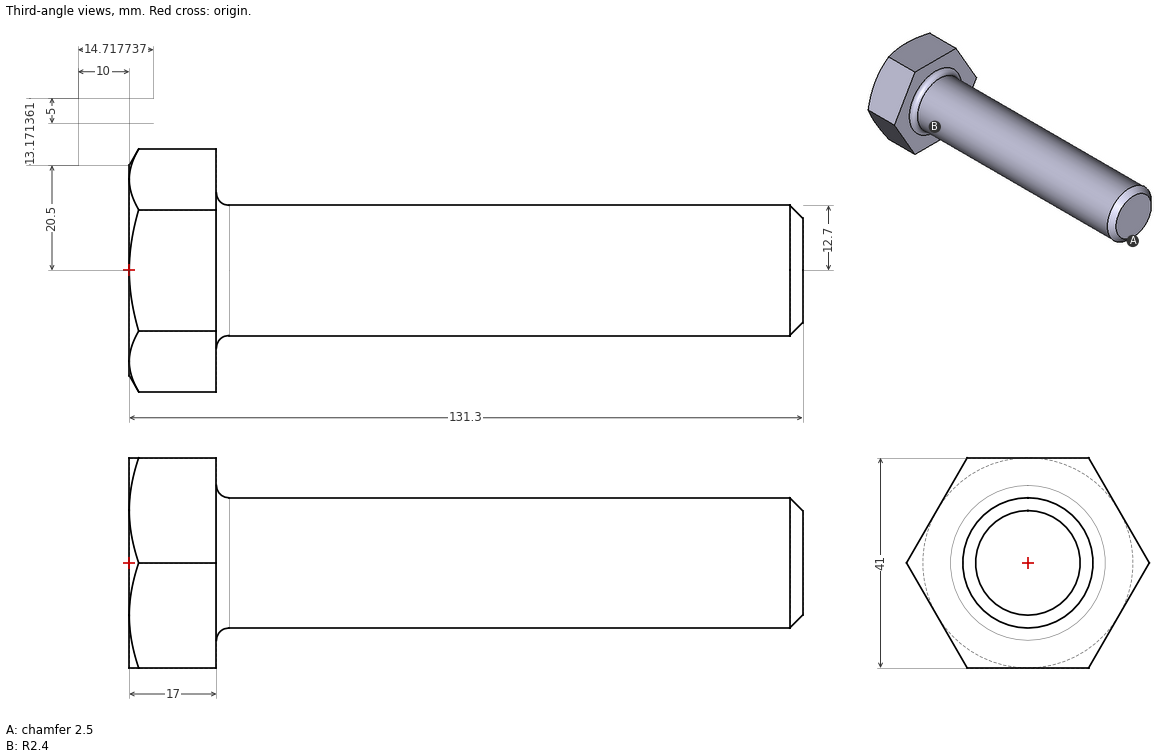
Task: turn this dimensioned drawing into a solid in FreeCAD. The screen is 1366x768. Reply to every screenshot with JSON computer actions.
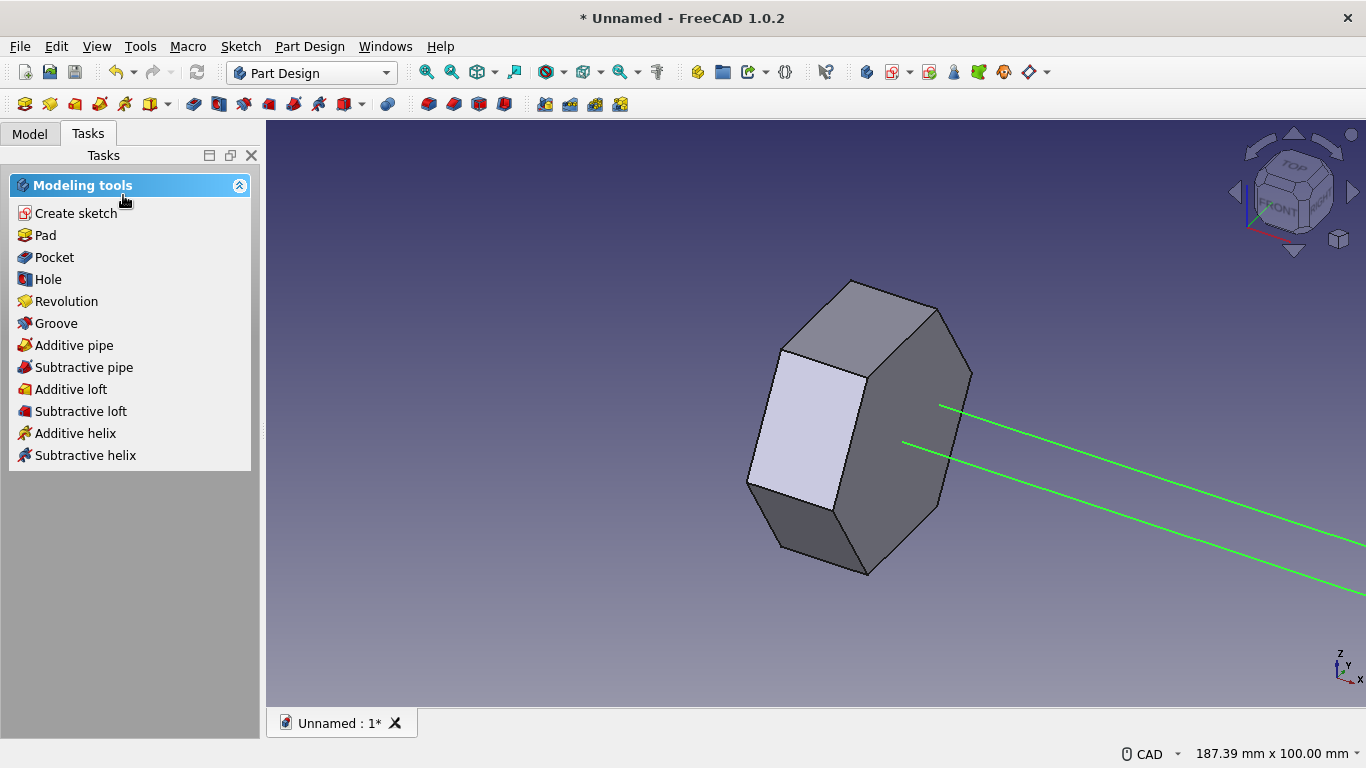
{"action": "left_click", "coordinate": [50, 104]}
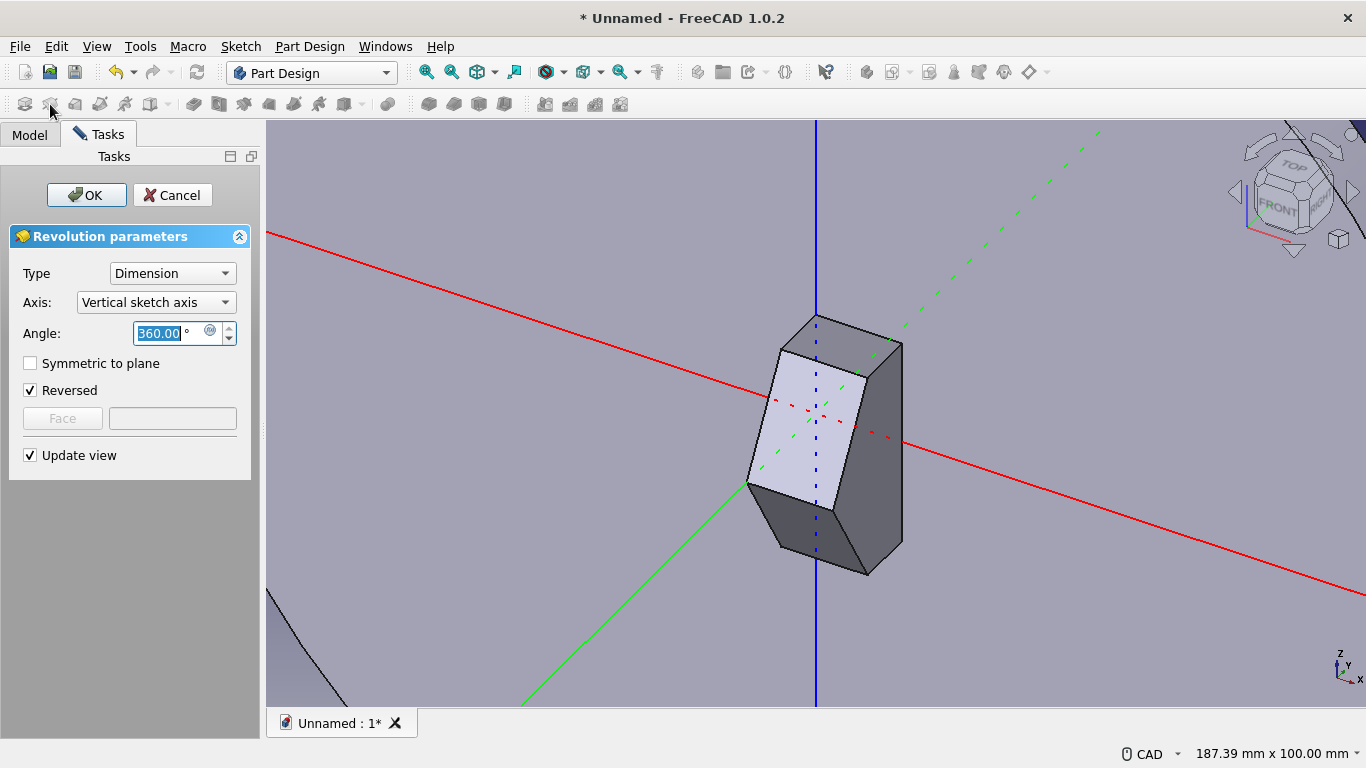
{"action": "left_click", "coordinate": [157, 302]}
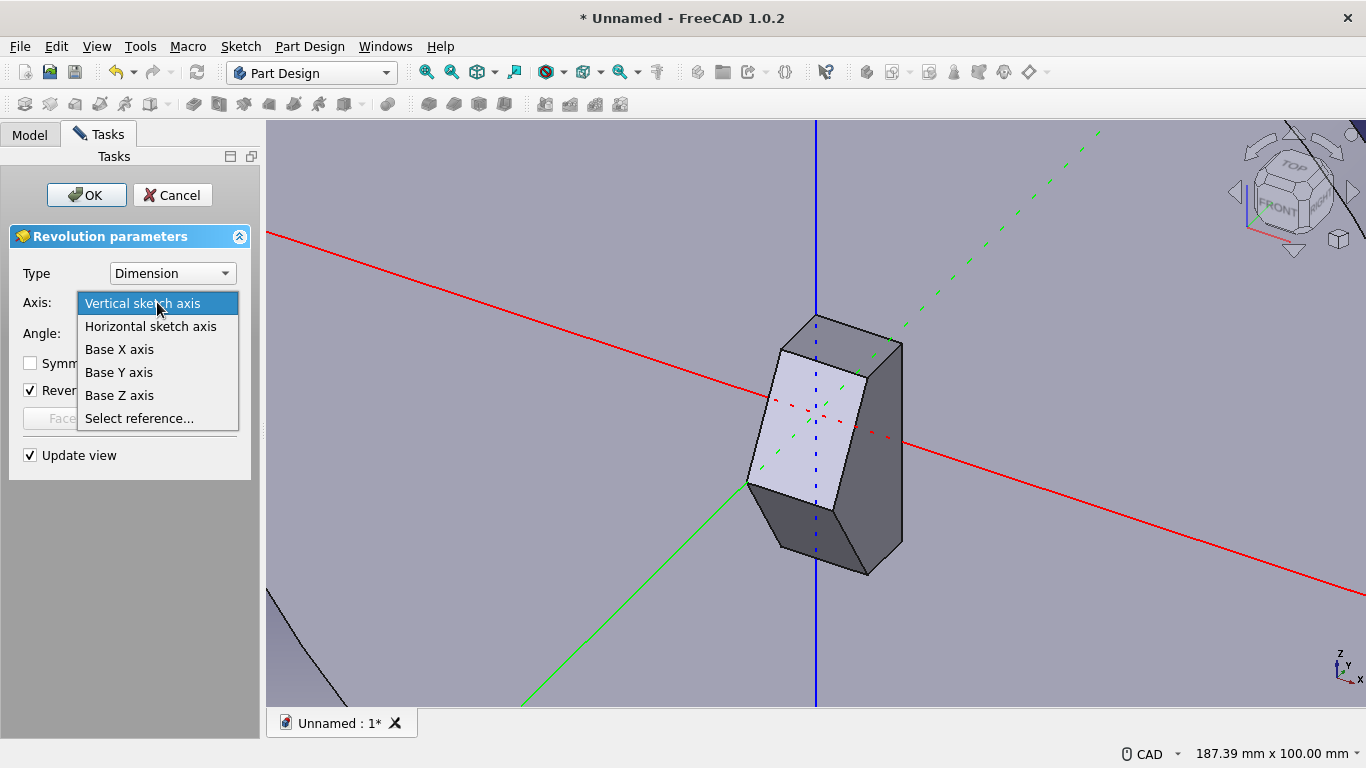
{"action": "left_click", "coordinate": [156, 326]}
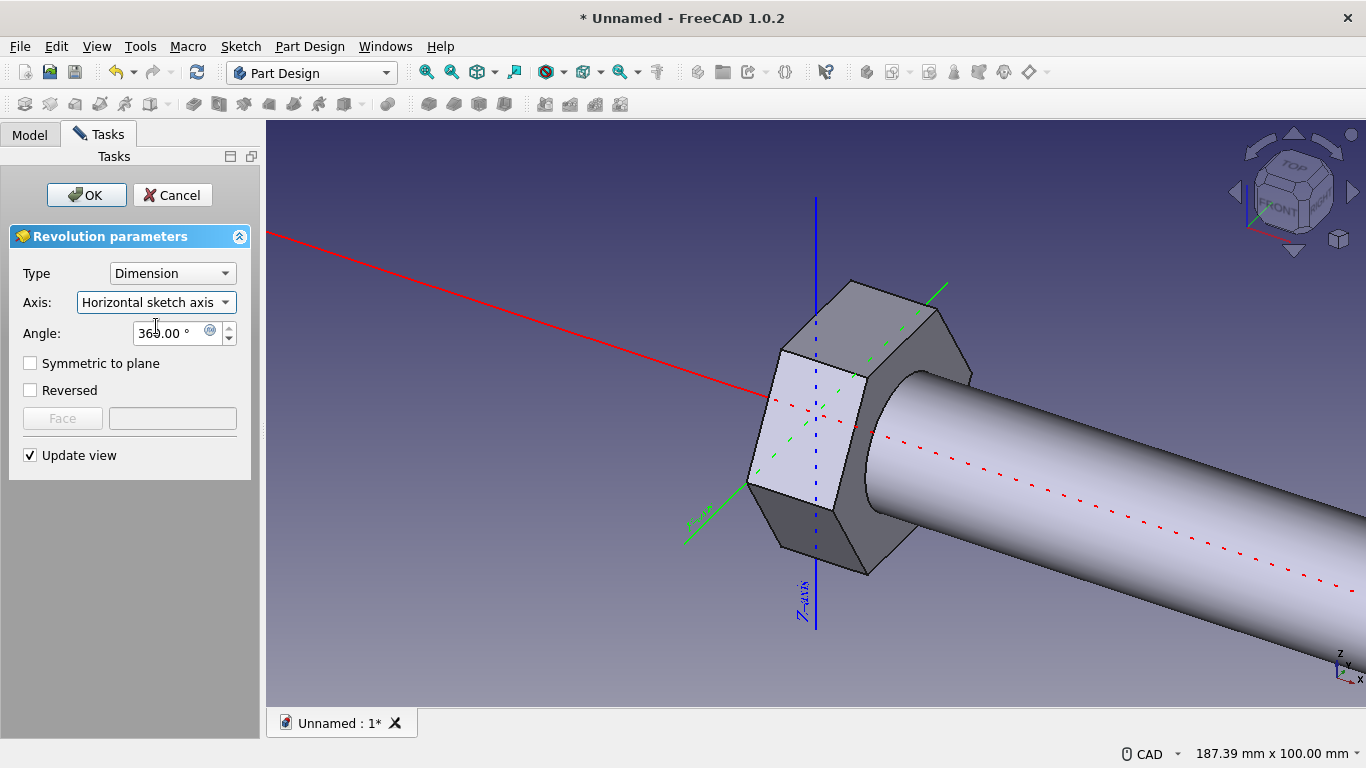
{"action": "left_click", "coordinate": [87, 195]}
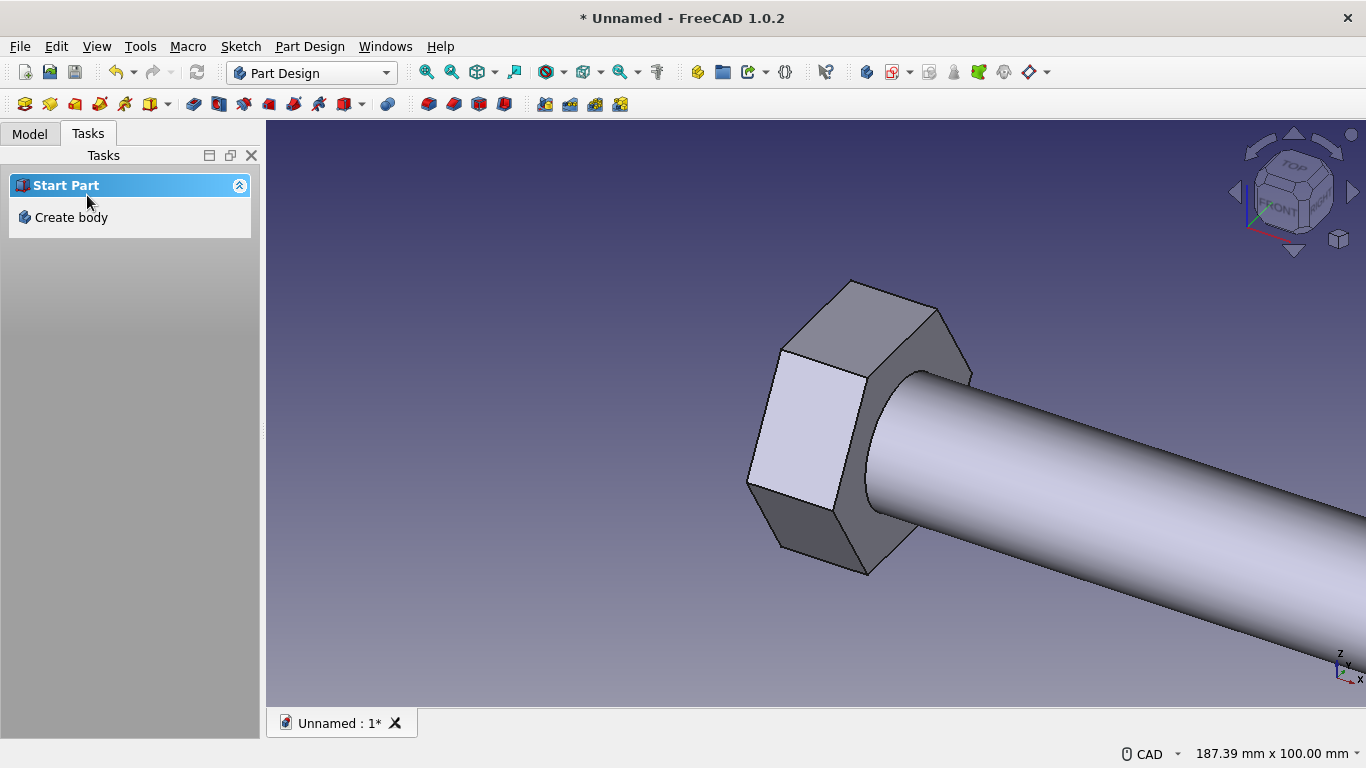
{"action": "key", "text": "v f"}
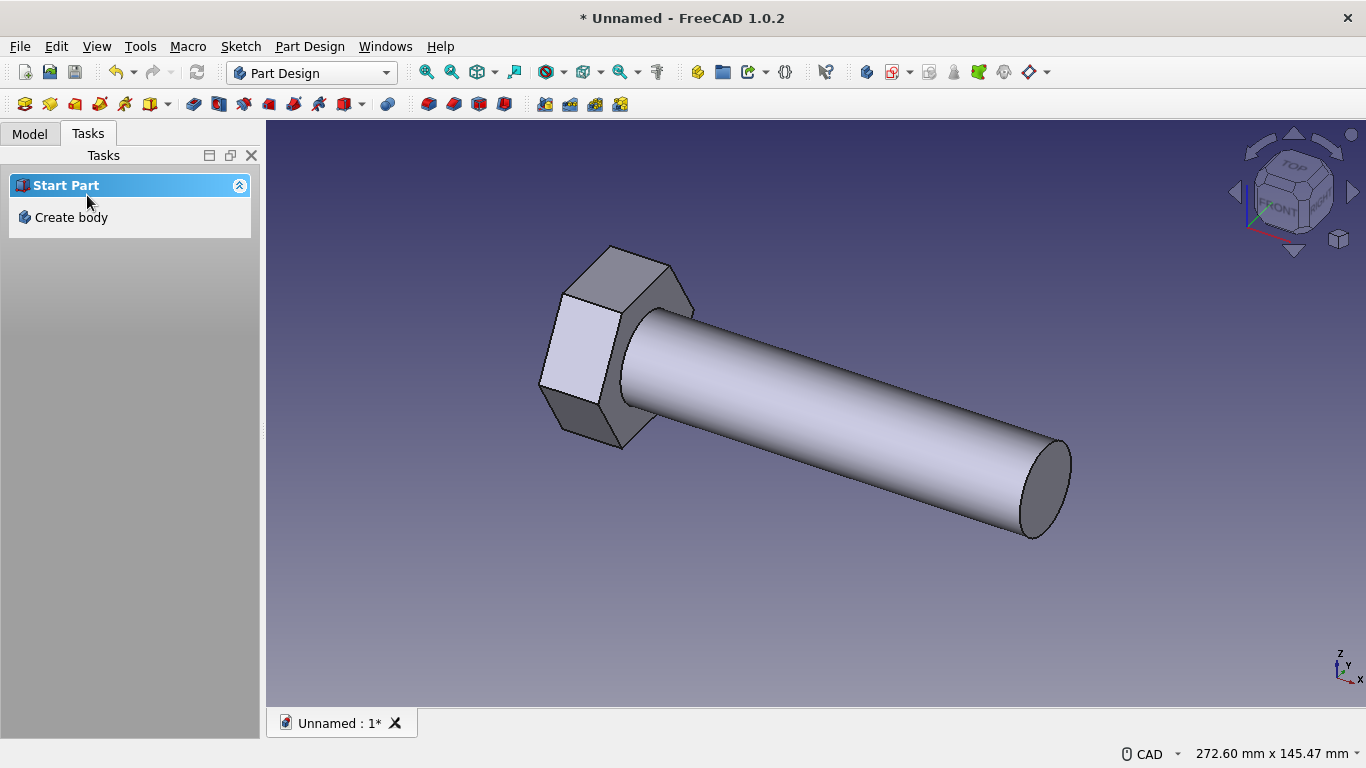
{"action": "left_click", "coordinate": [892, 72]}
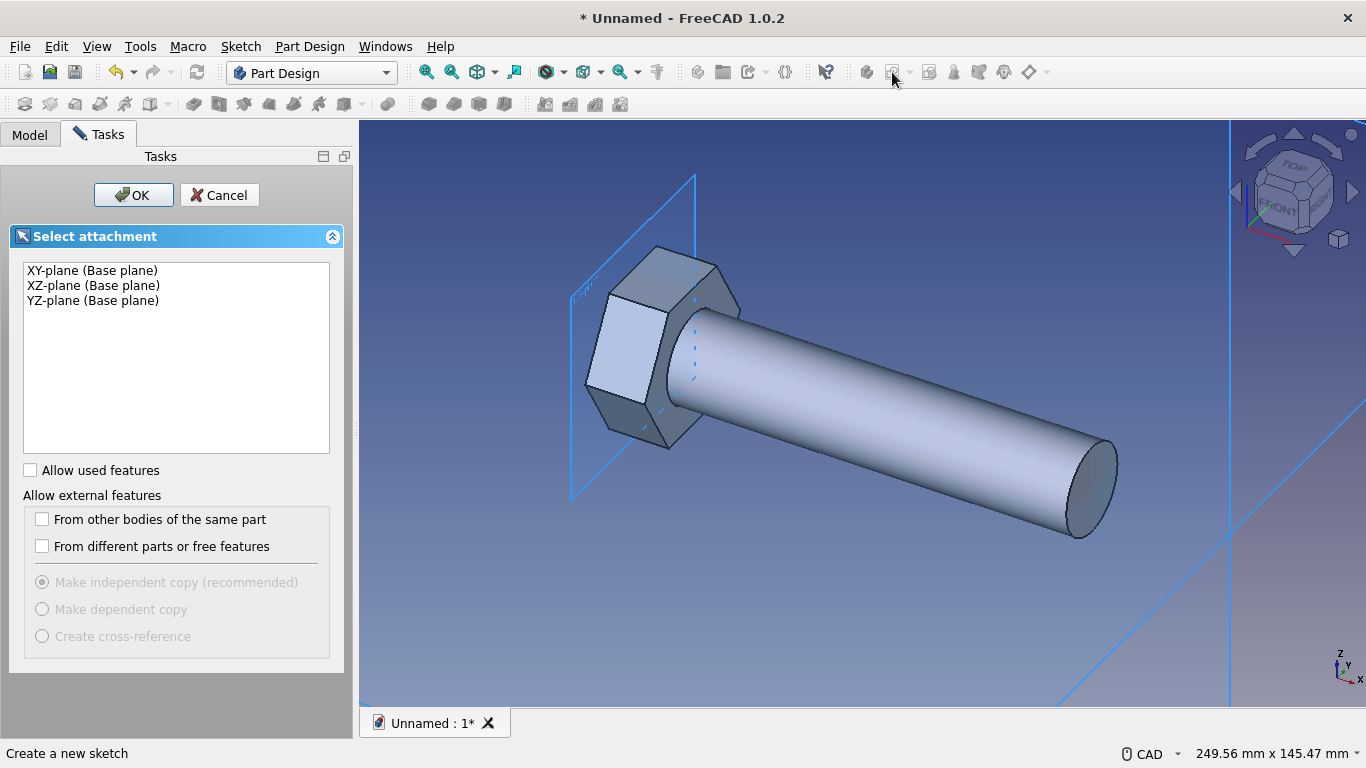
{"action": "left_click", "coordinate": [84, 270]}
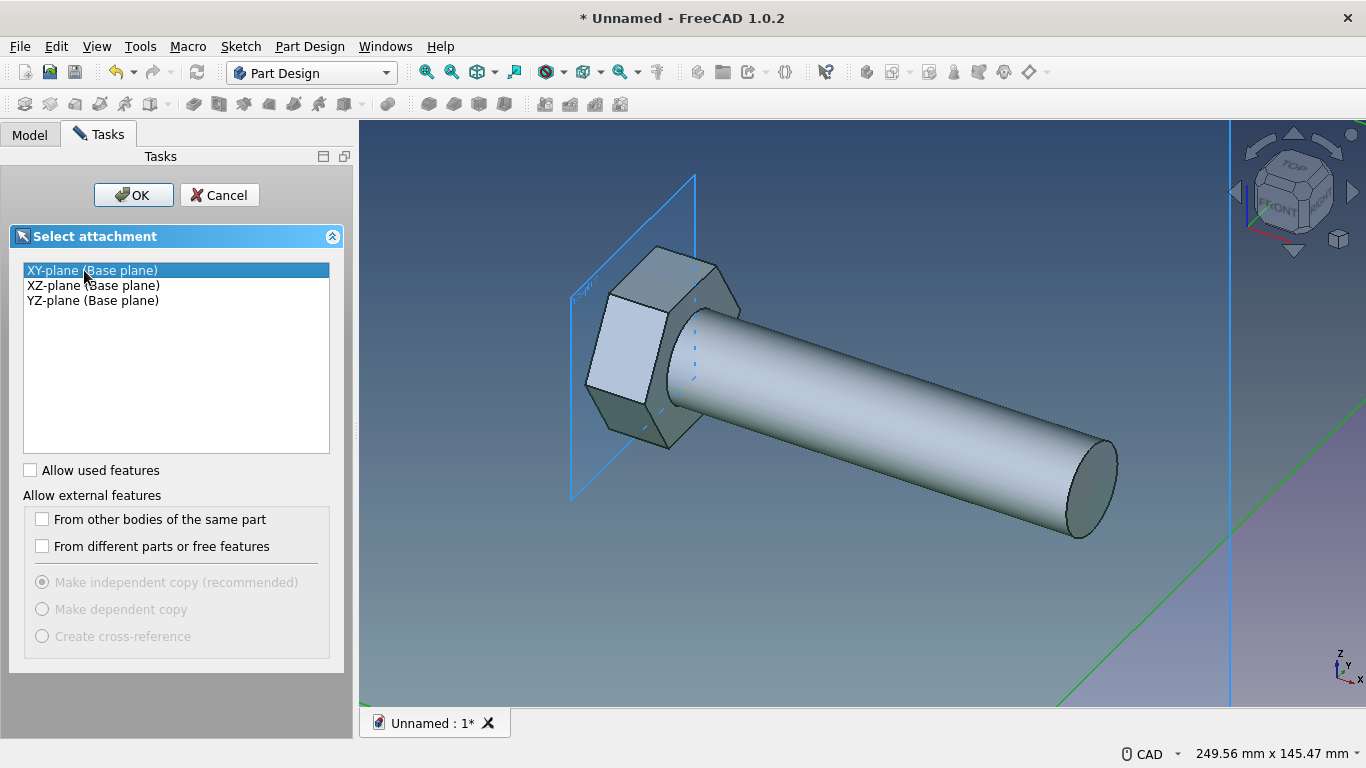
{"action": "left_click", "coordinate": [134, 195]}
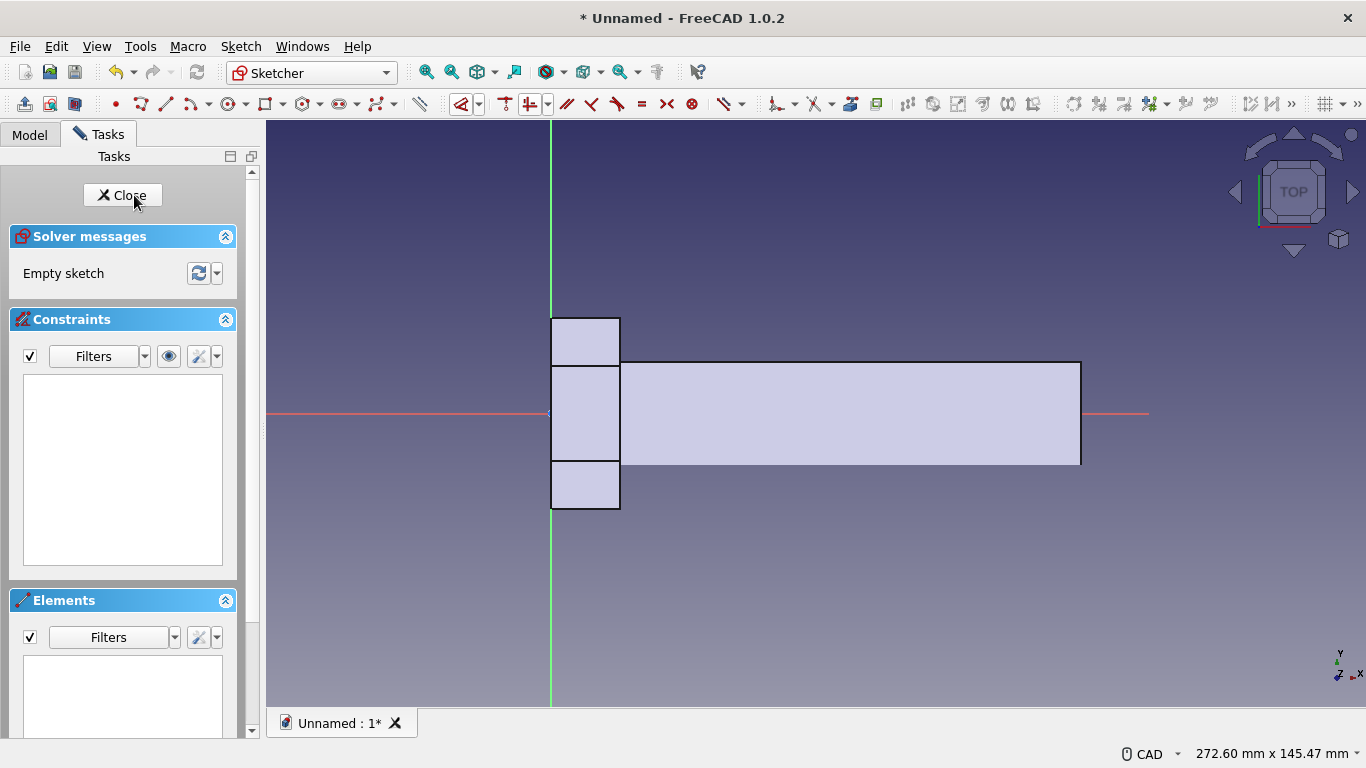
{"action": "key", "text": "q s"}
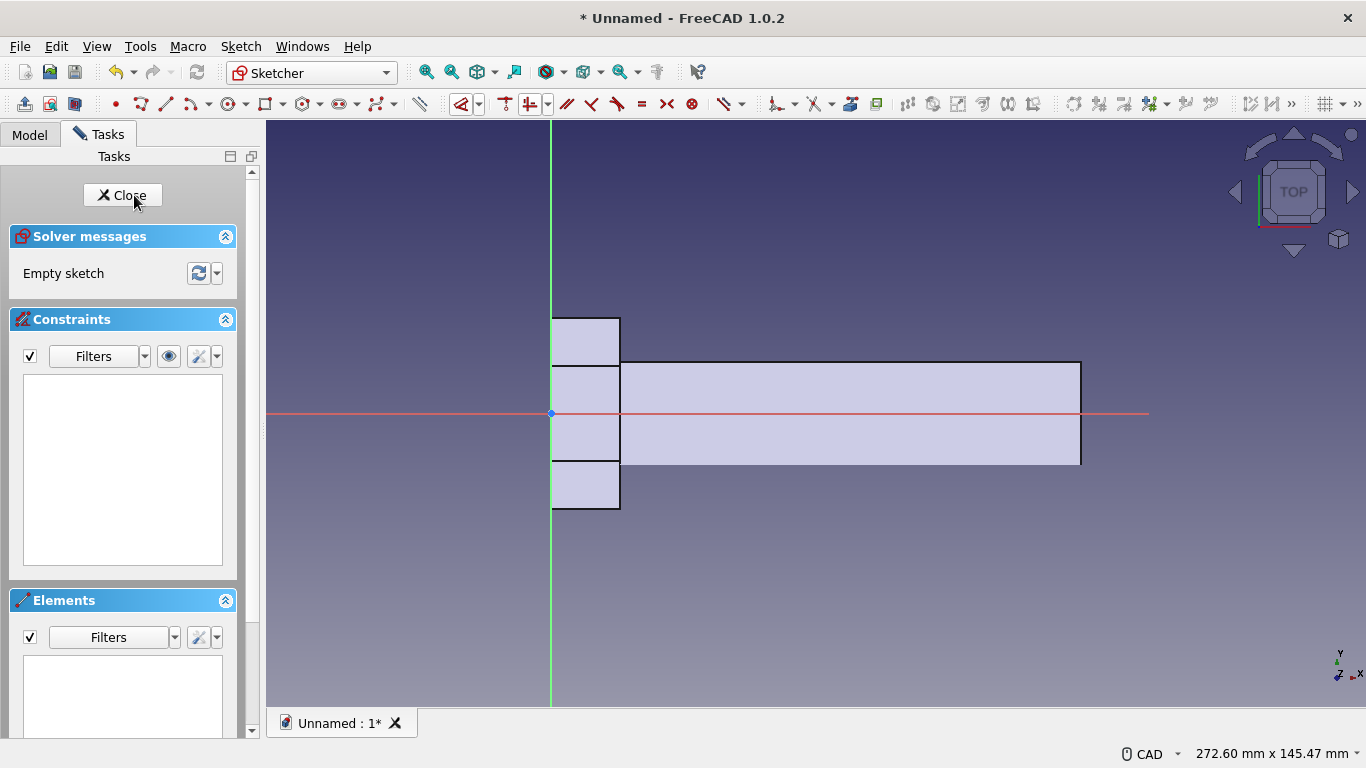
{"action": "scroll", "coordinate": [420, 306], "scroll_direction": "up", "scroll_amount": 5}